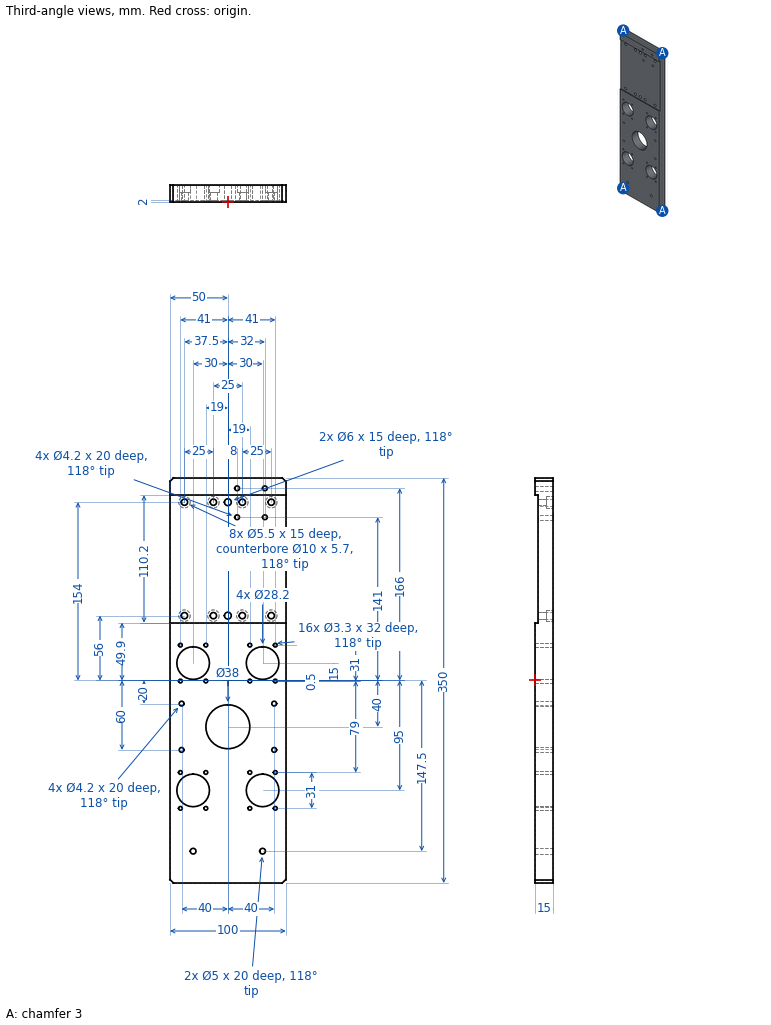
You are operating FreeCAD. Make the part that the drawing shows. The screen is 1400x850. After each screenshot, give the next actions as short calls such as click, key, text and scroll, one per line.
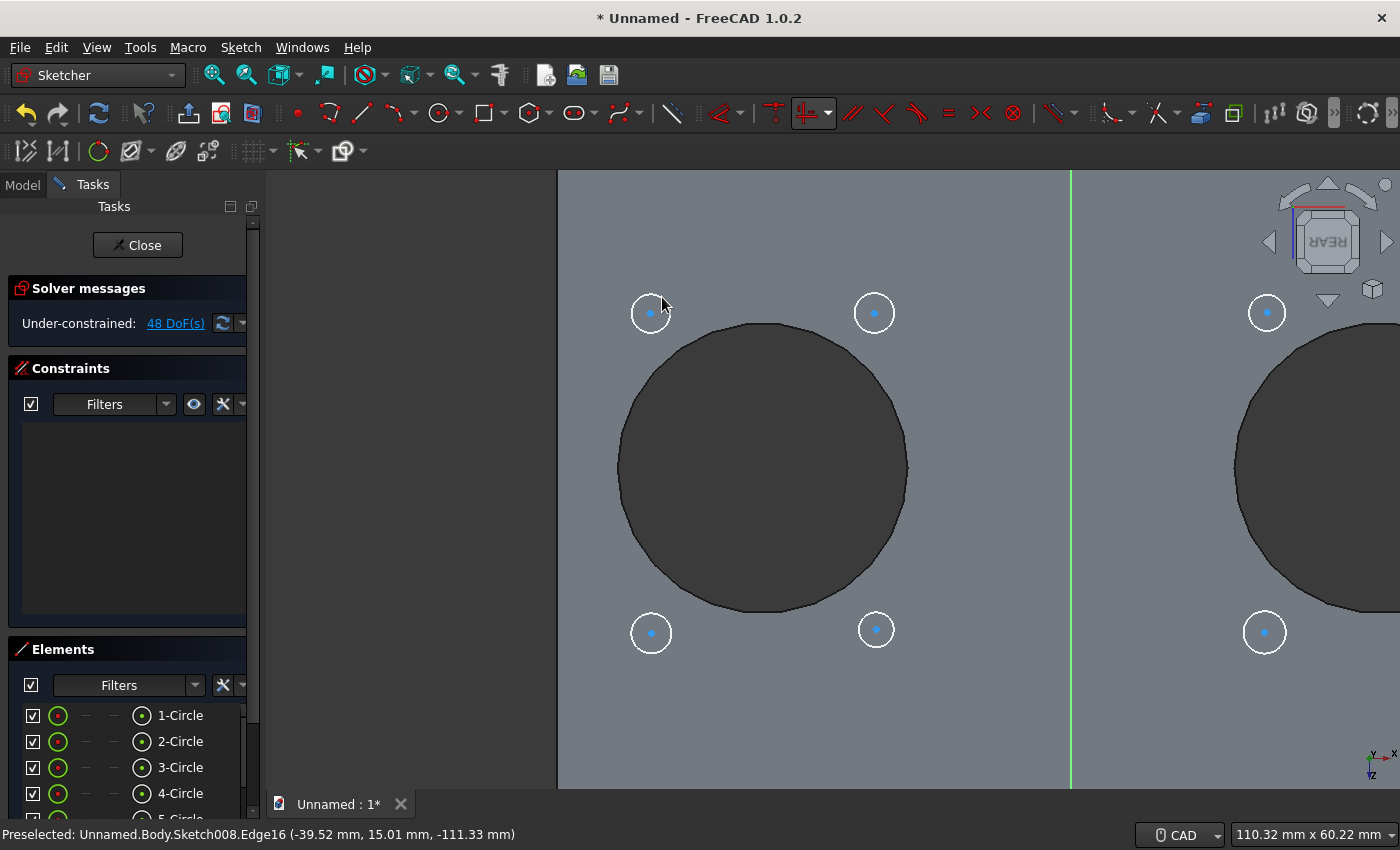
scroll(664, 298, down, 7)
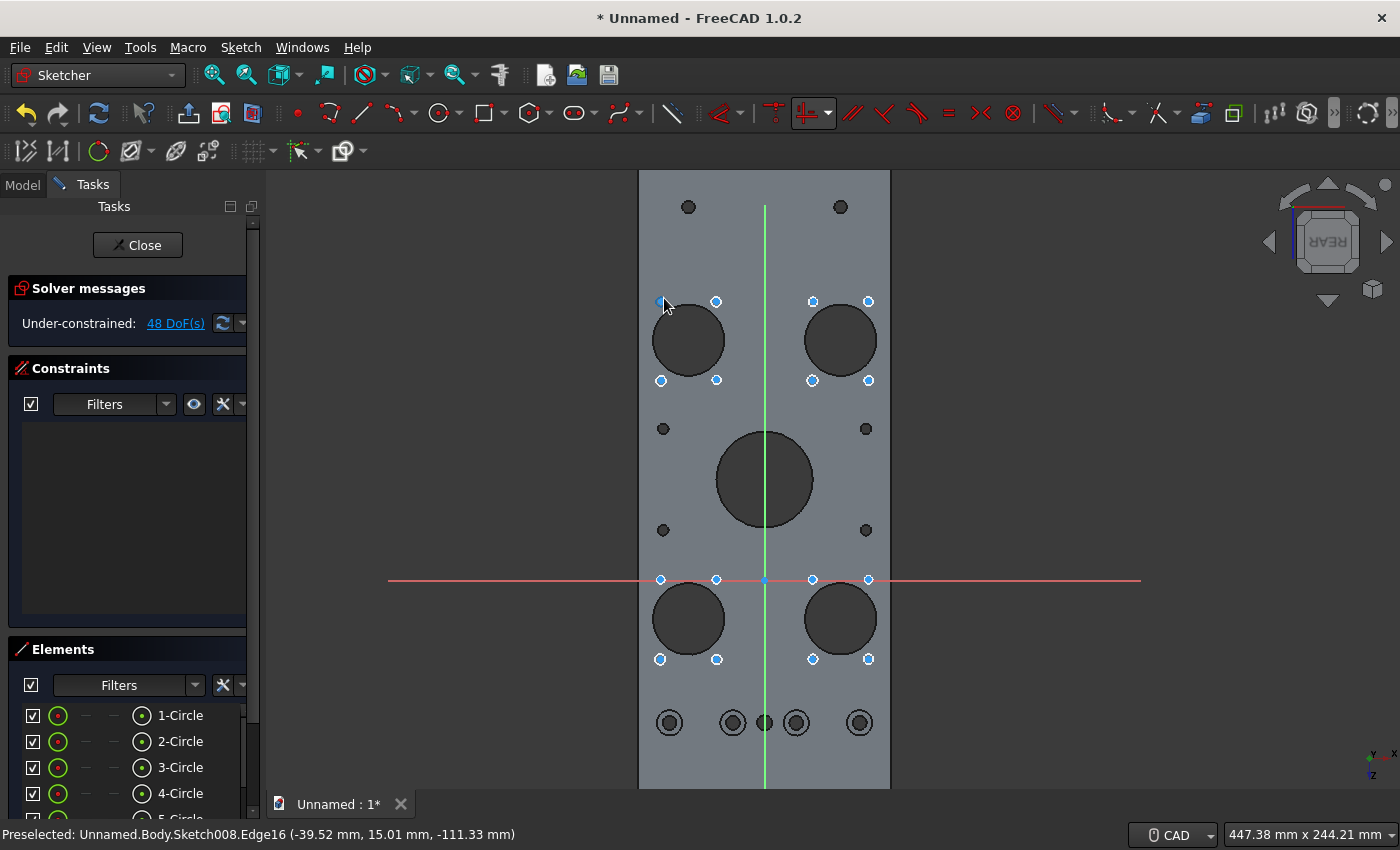
scroll(872, 656, up, 6)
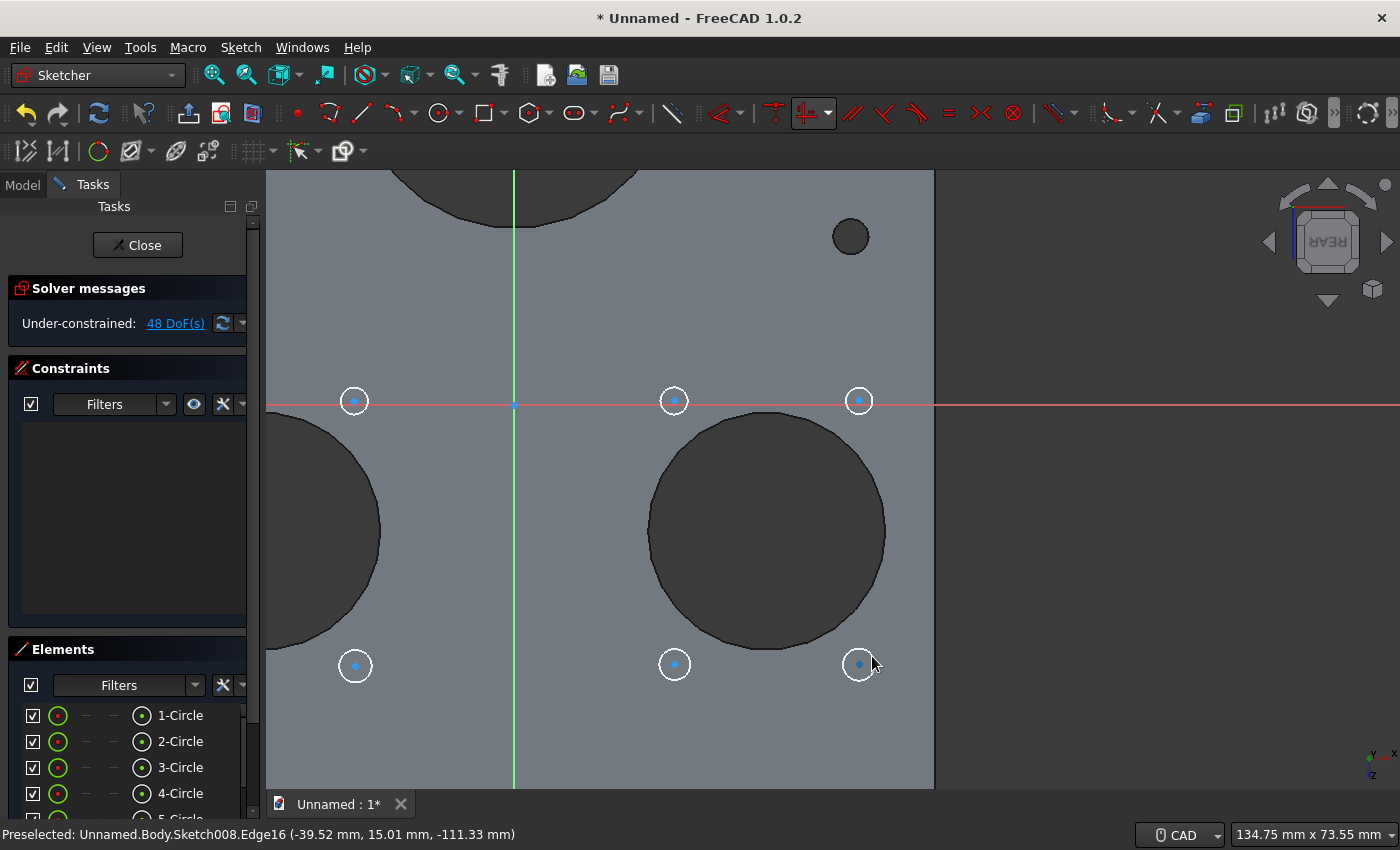
click(870, 653)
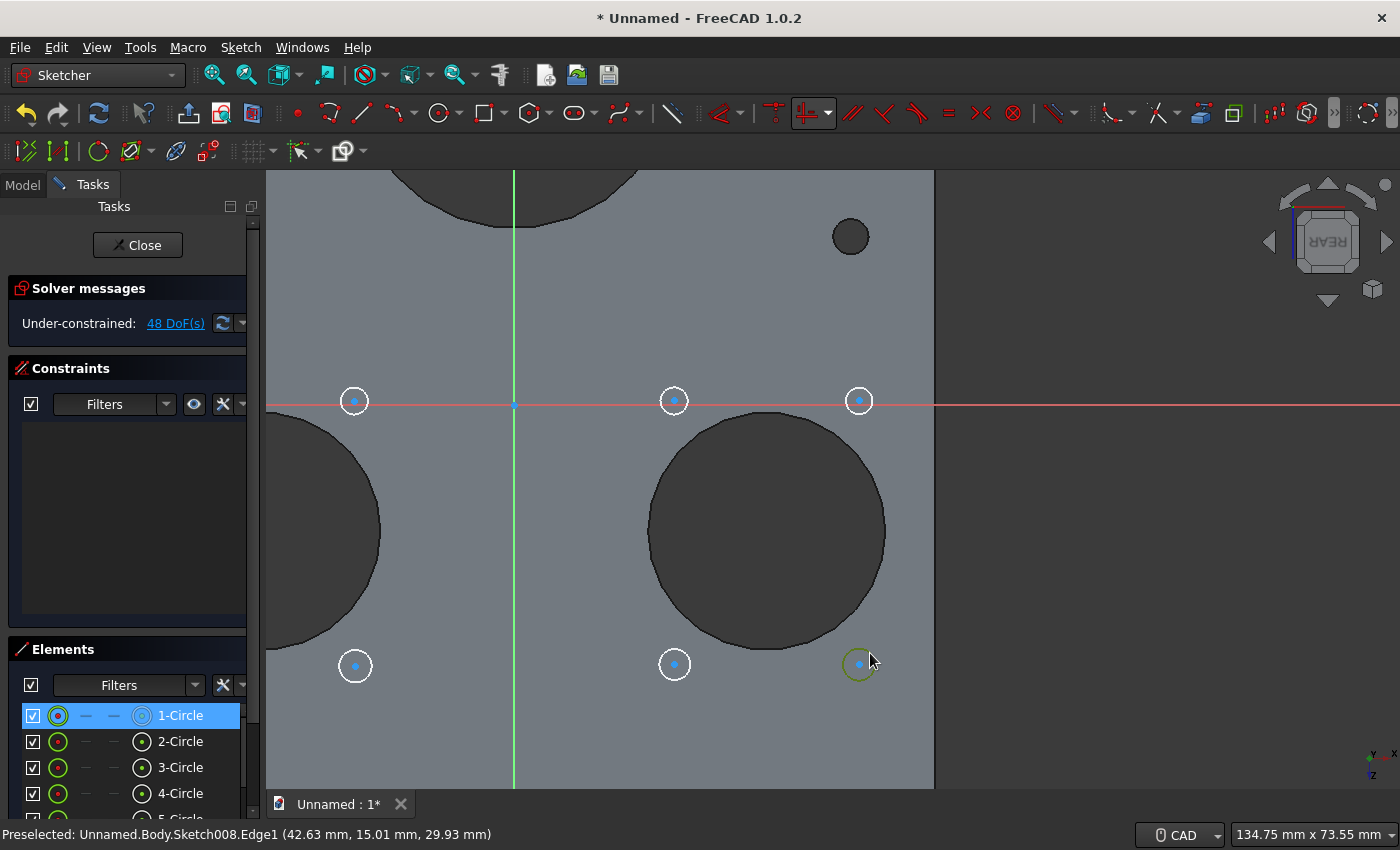
click(686, 654)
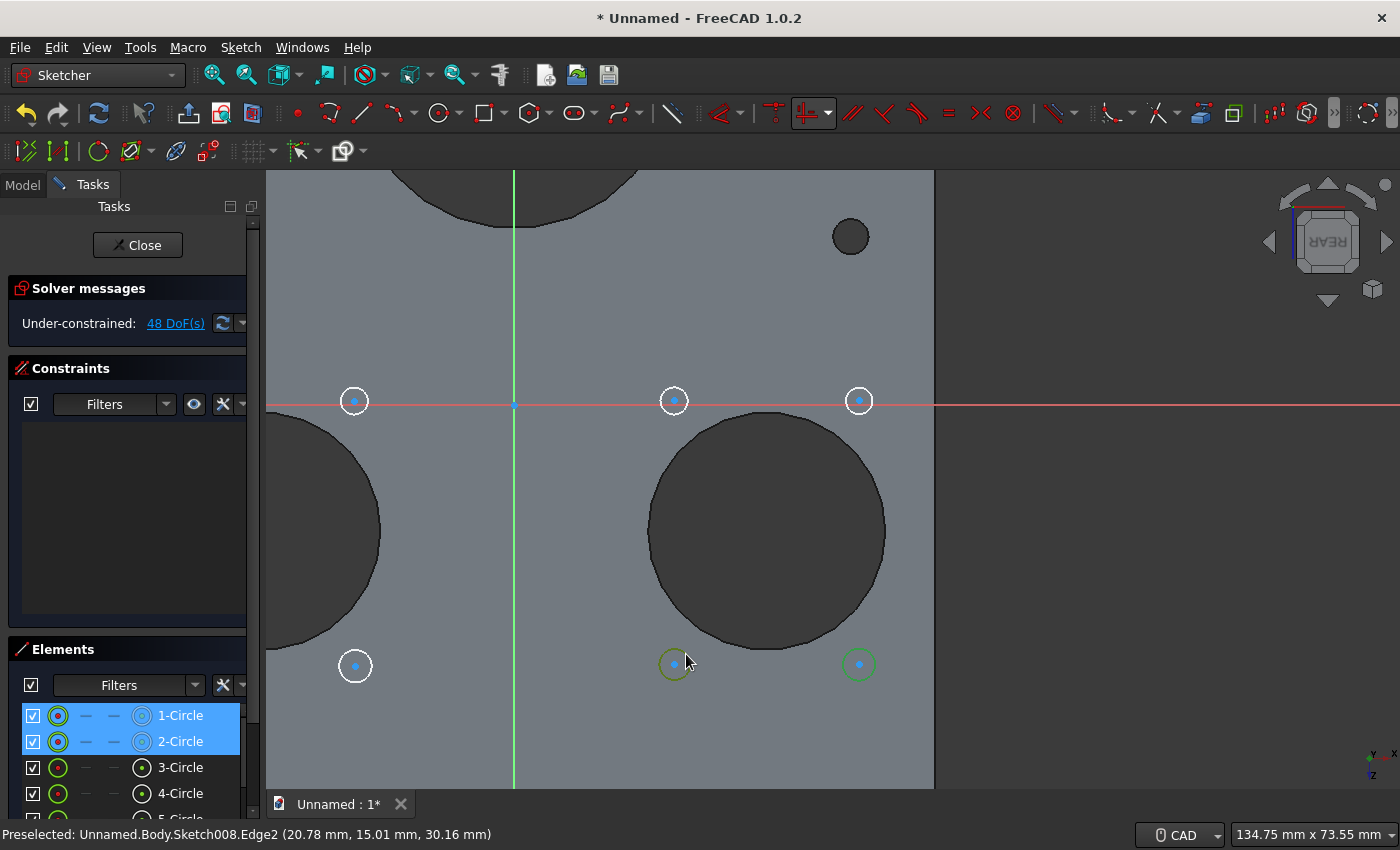
click(869, 392)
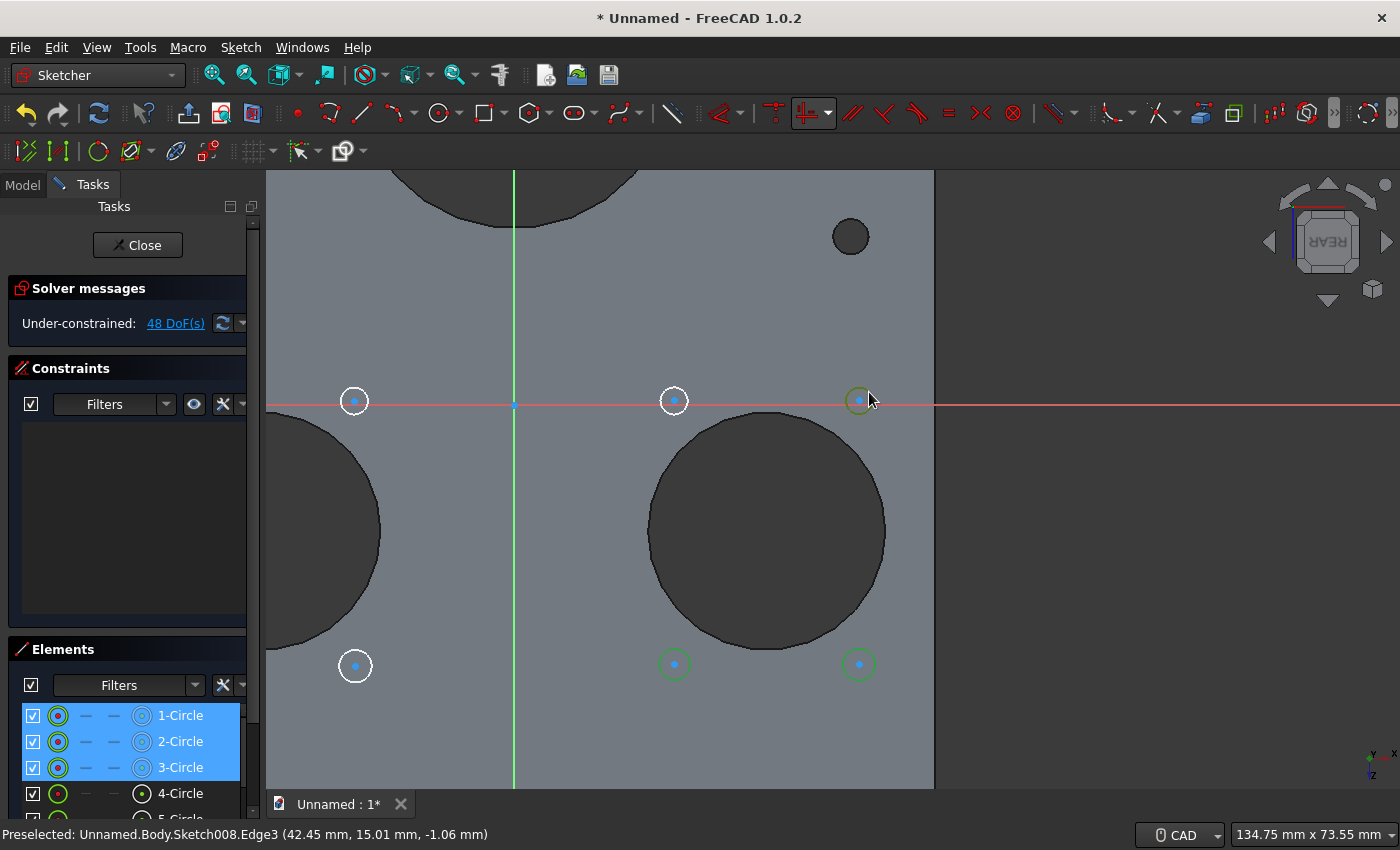
click(684, 391)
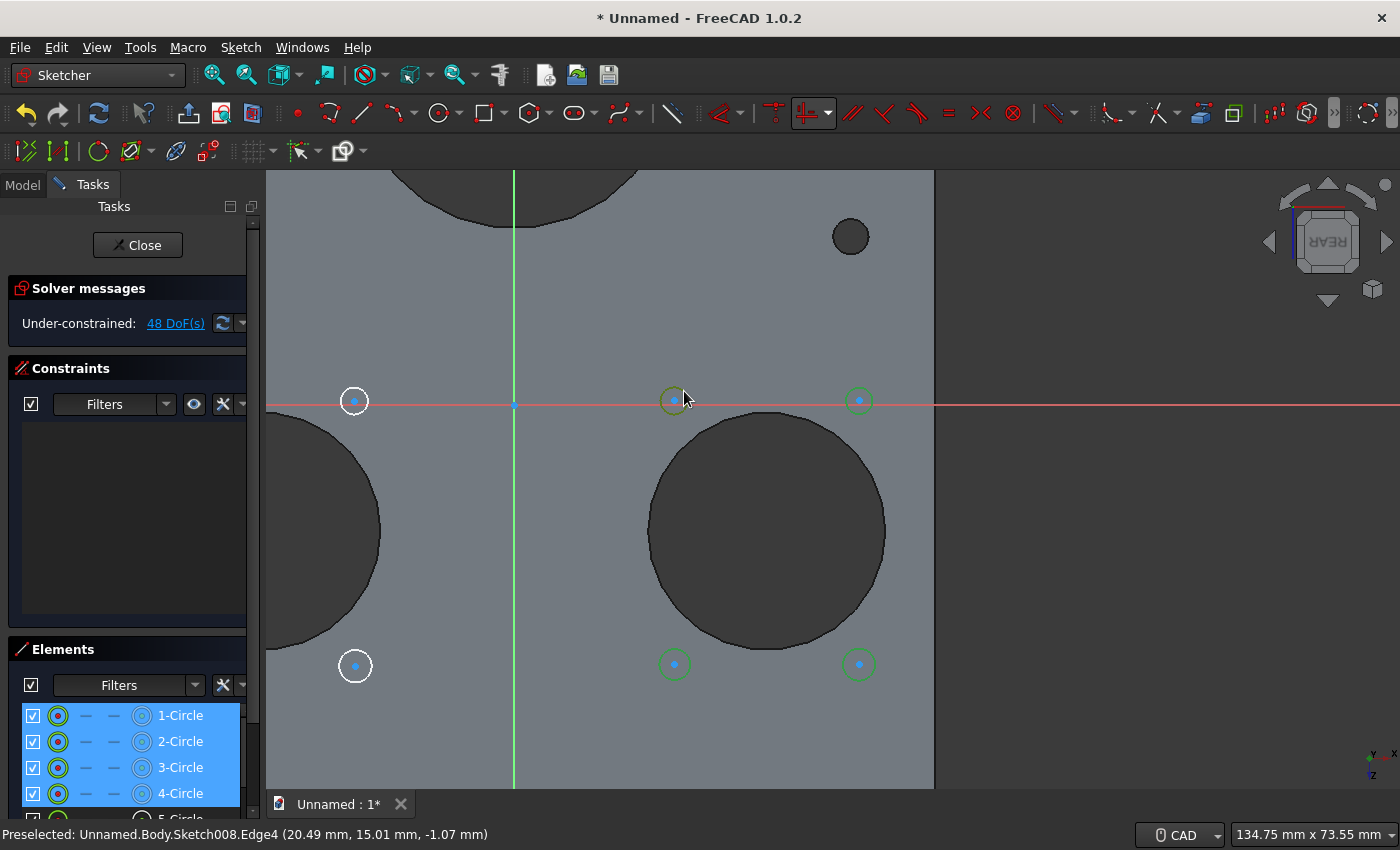
click(367, 655)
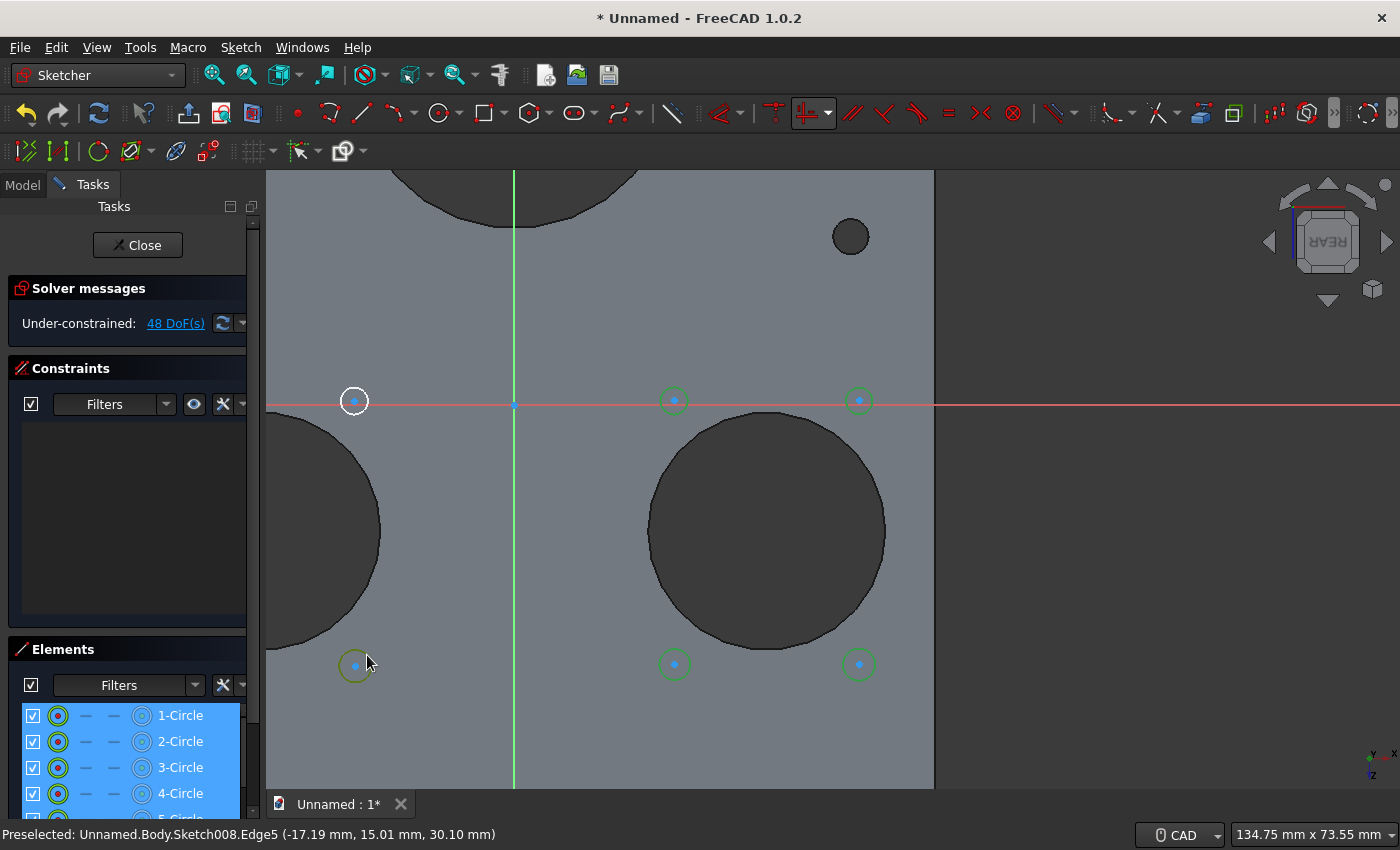
scroll(872, 657, down, 6)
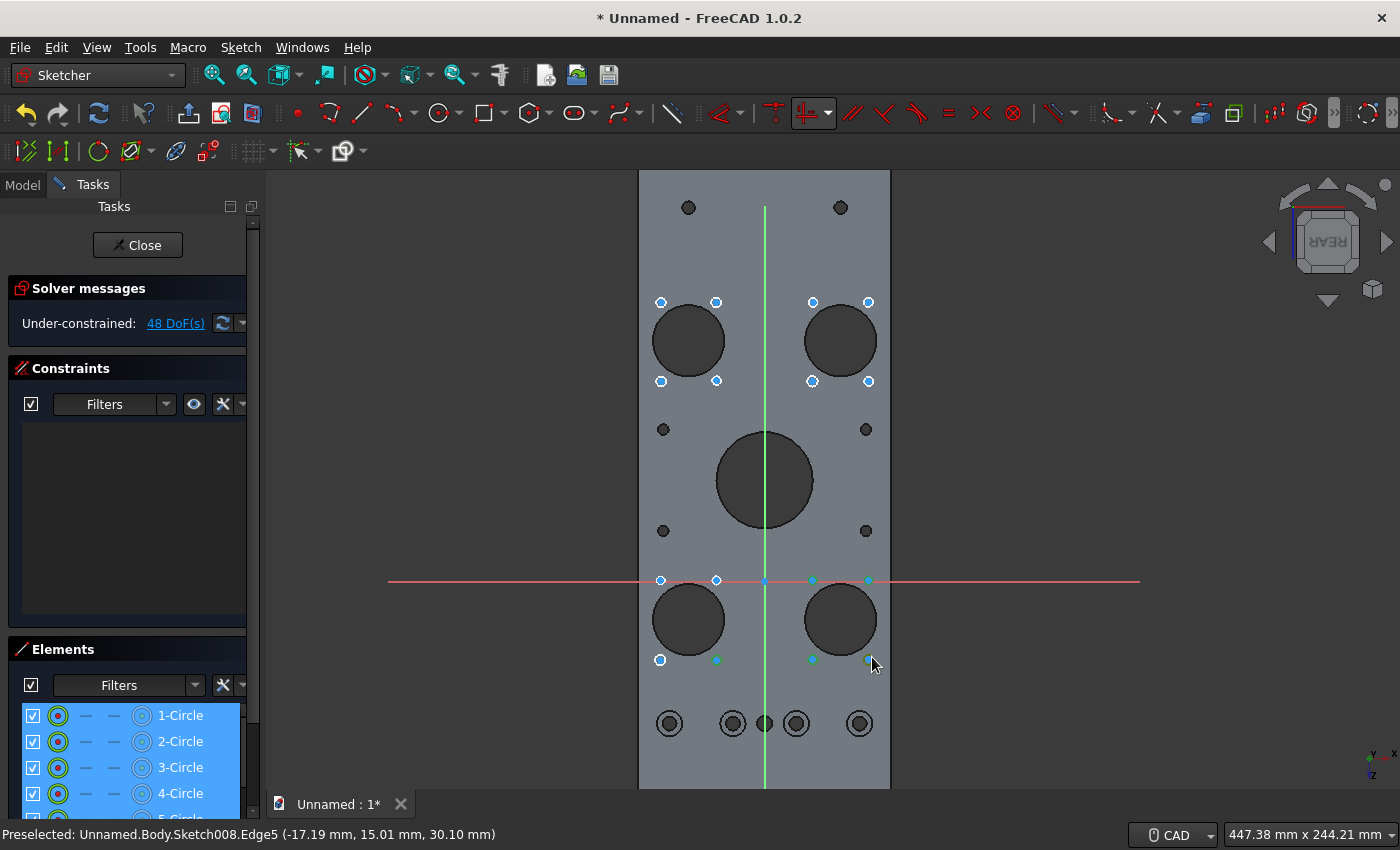
scroll(664, 656, up, 5)